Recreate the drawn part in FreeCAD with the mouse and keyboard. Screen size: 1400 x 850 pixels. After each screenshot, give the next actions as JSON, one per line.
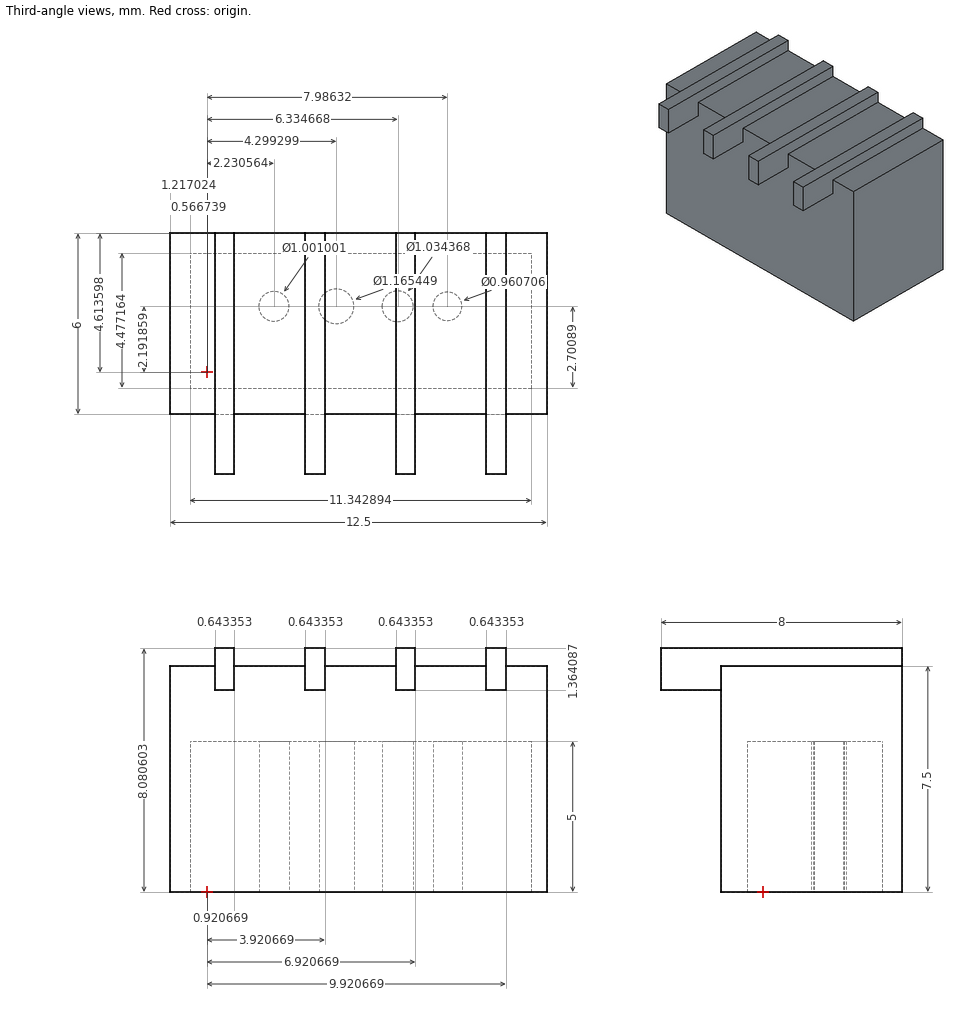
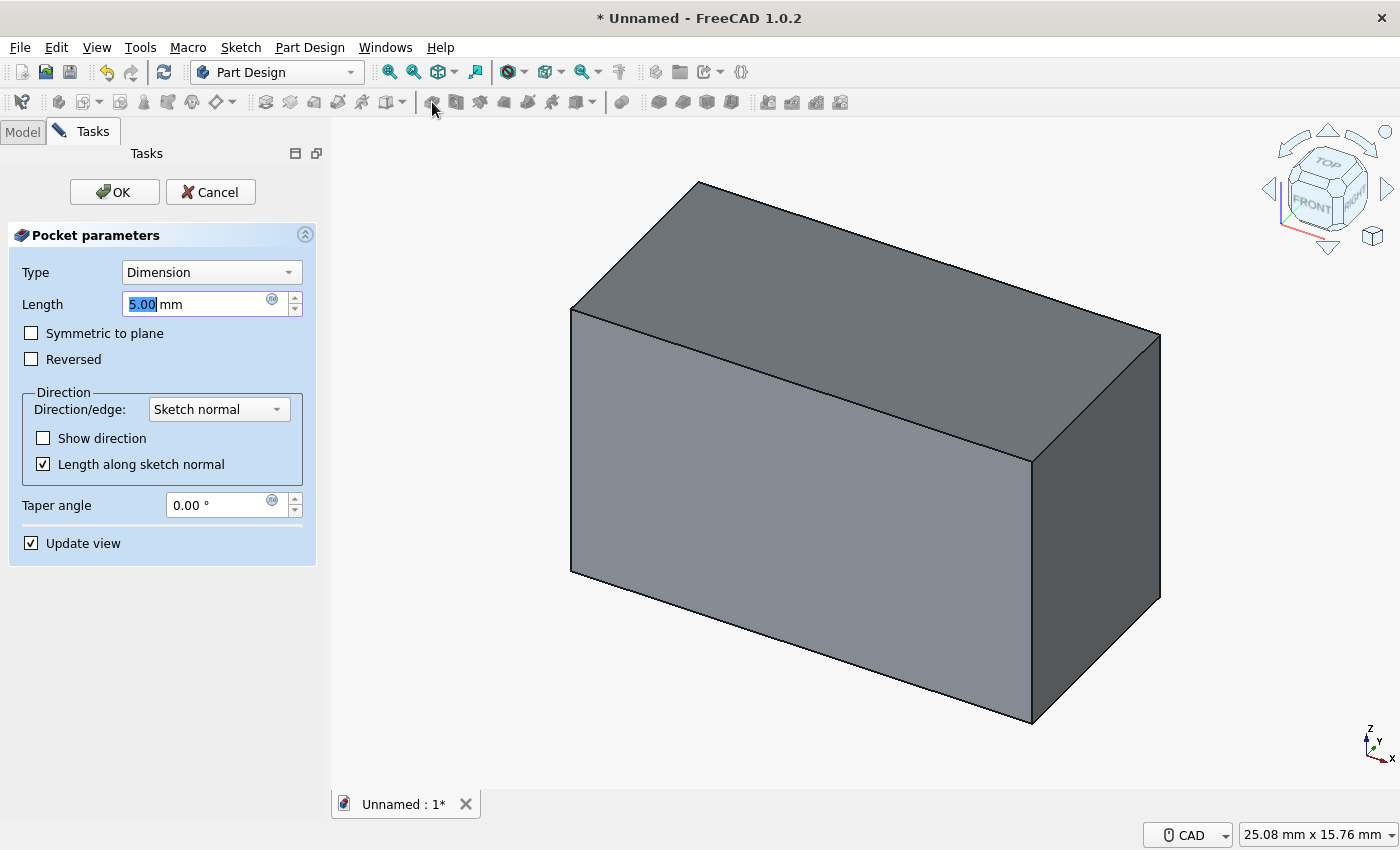
{"action": "type", "text": "5"}
{"action": "key", "text": "Tab"}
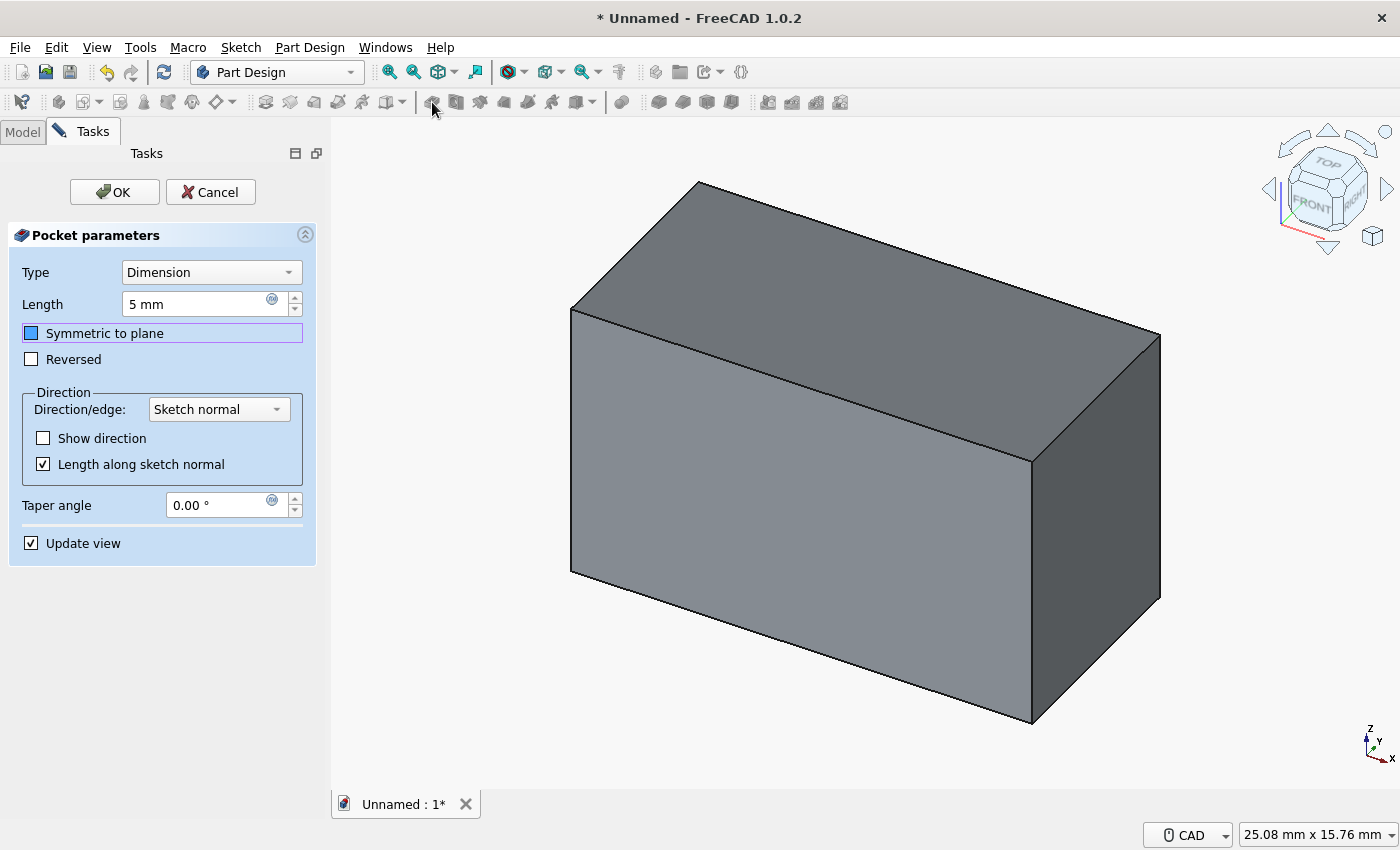
{"action": "left_click", "coordinate": [30, 359]}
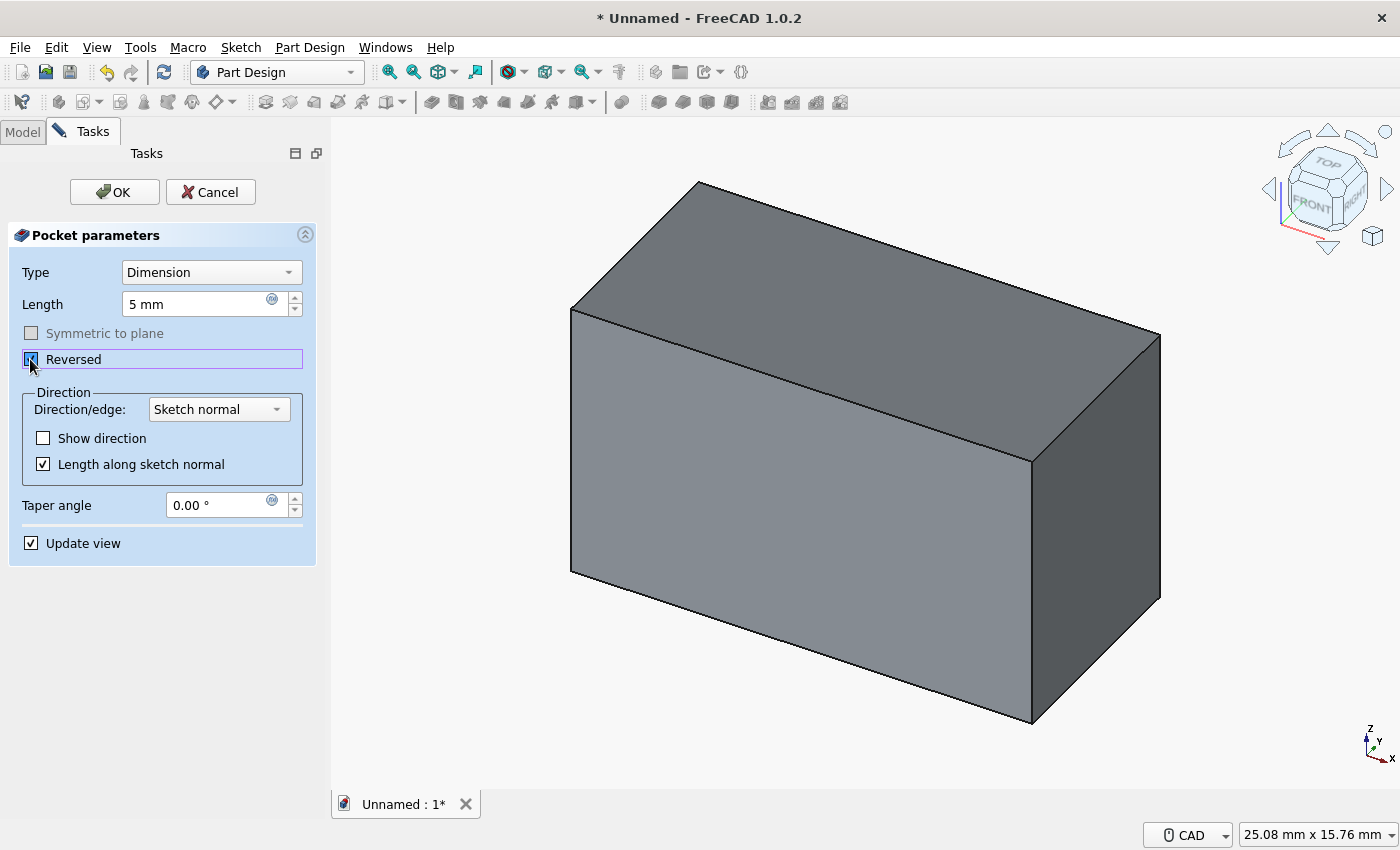
{"action": "left_click", "coordinate": [115, 192]}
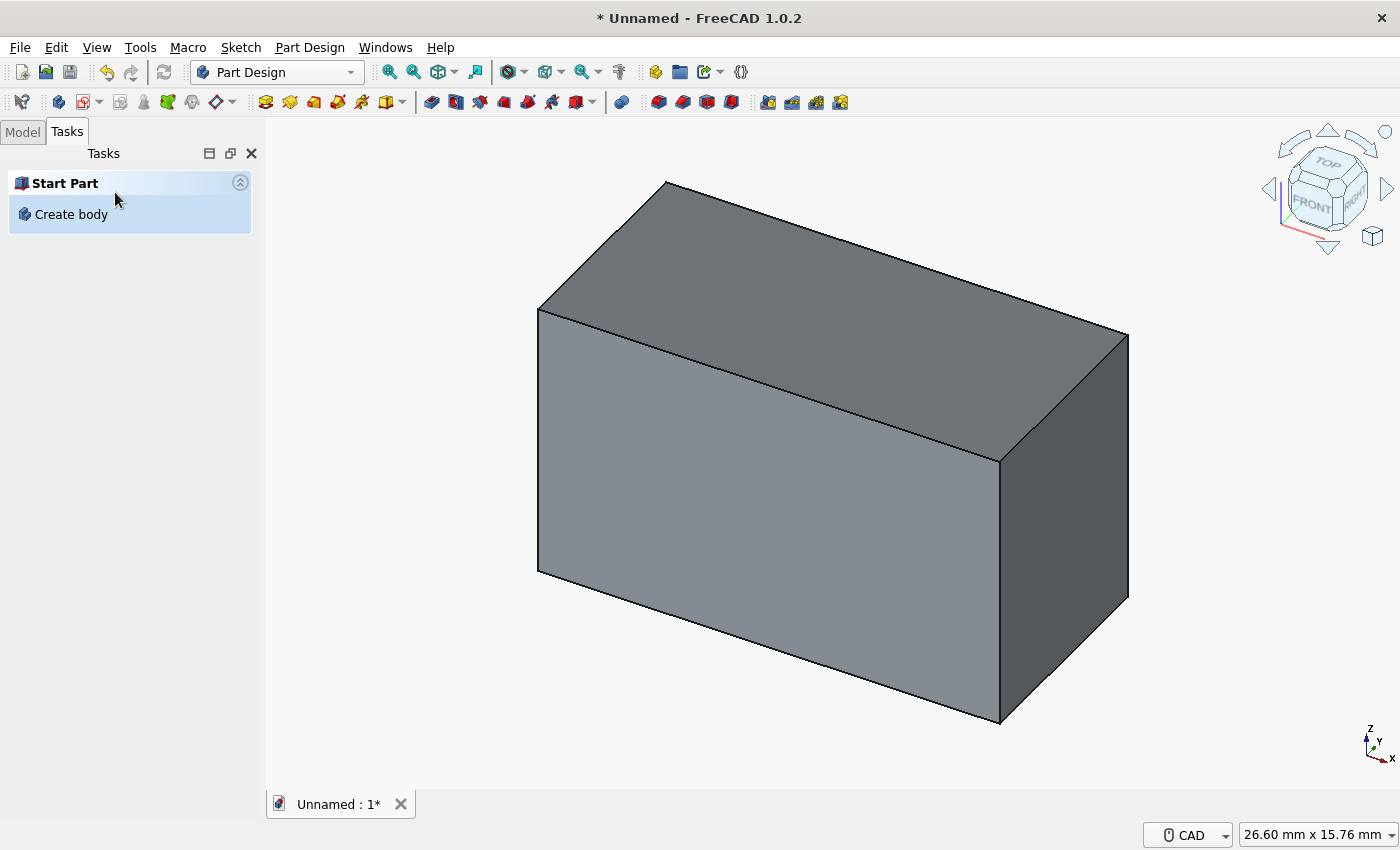
{"action": "key", "text": "4"}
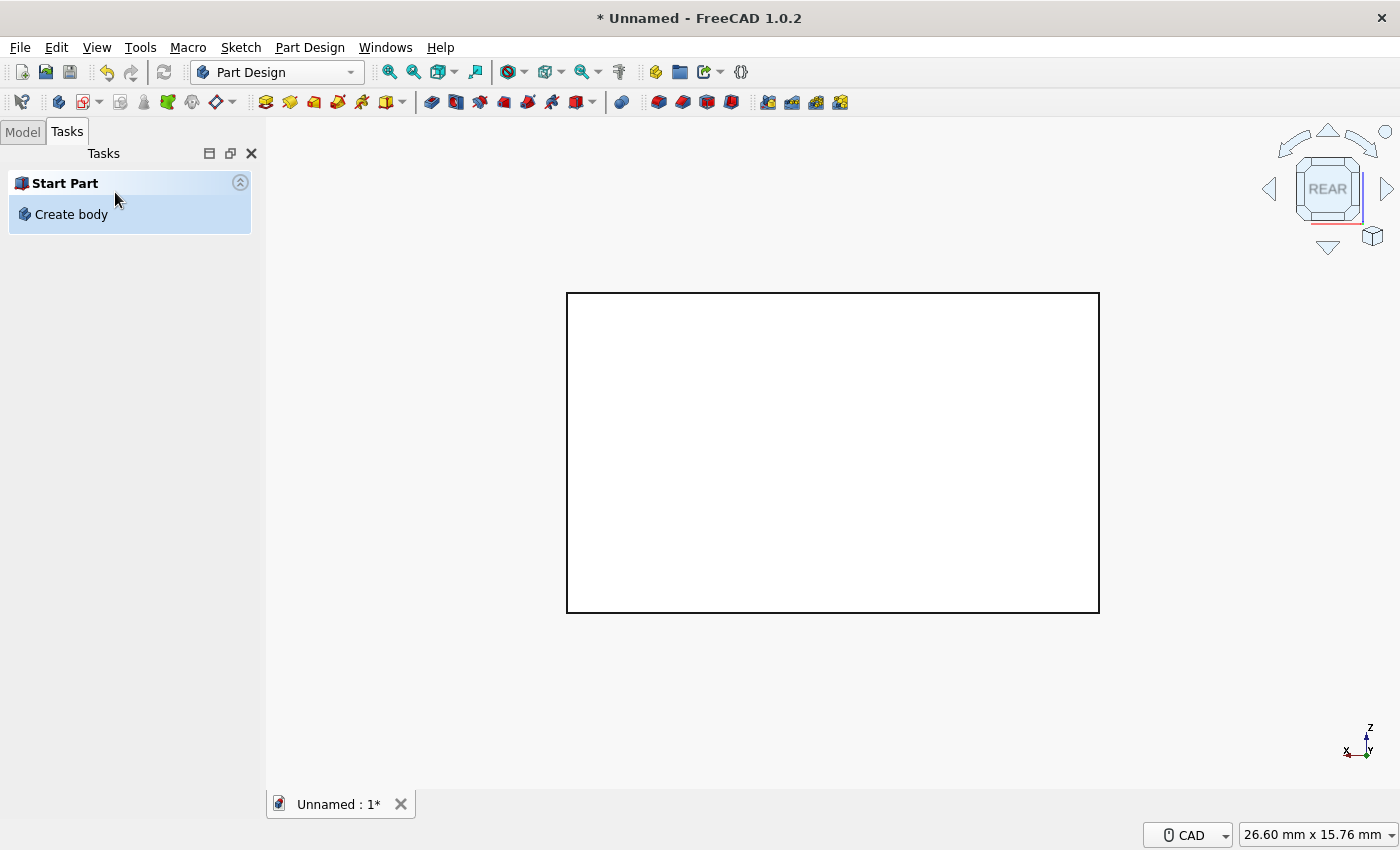
{"action": "left_click", "coordinate": [757, 452]}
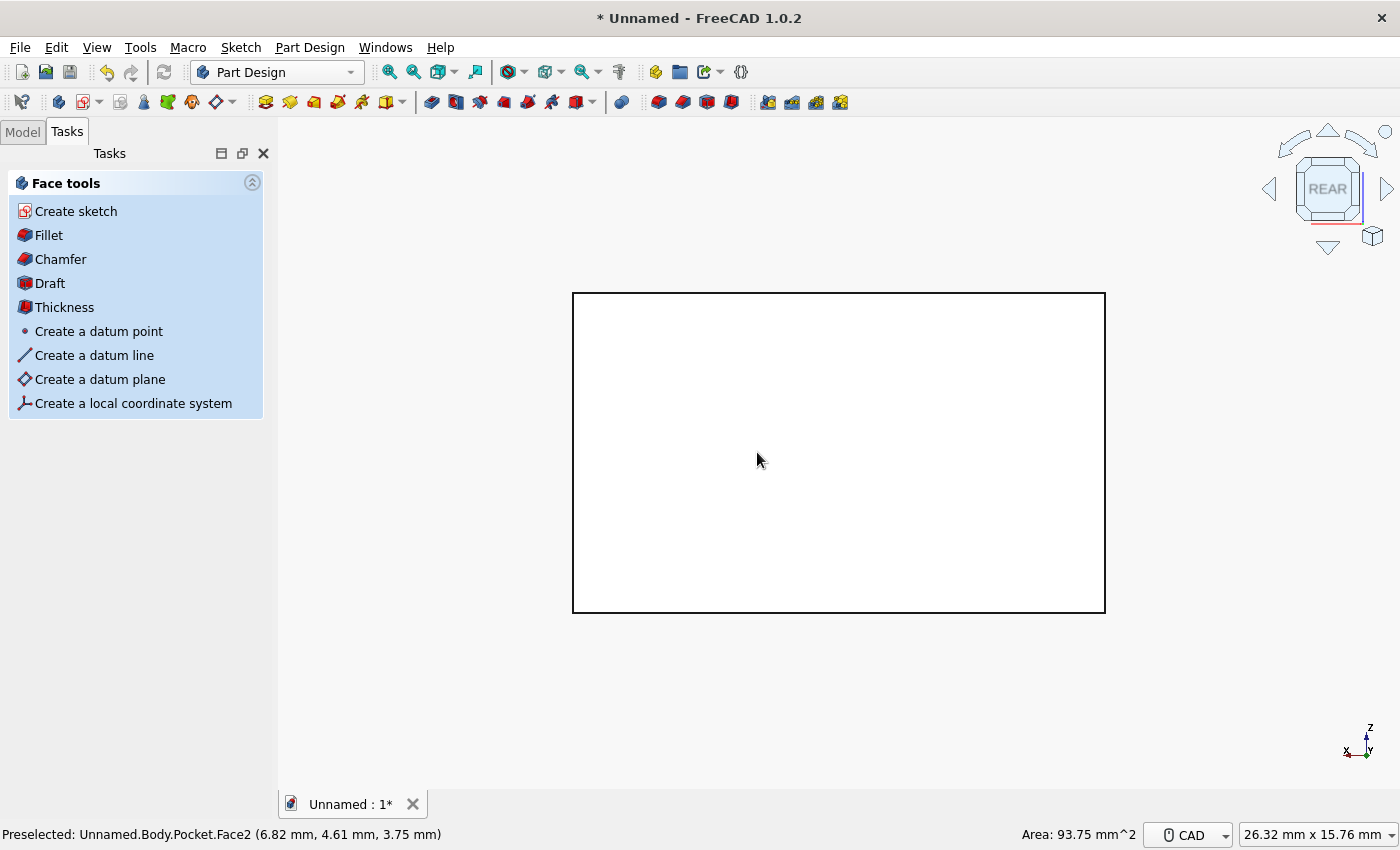
{"action": "left_click", "coordinate": [84, 102]}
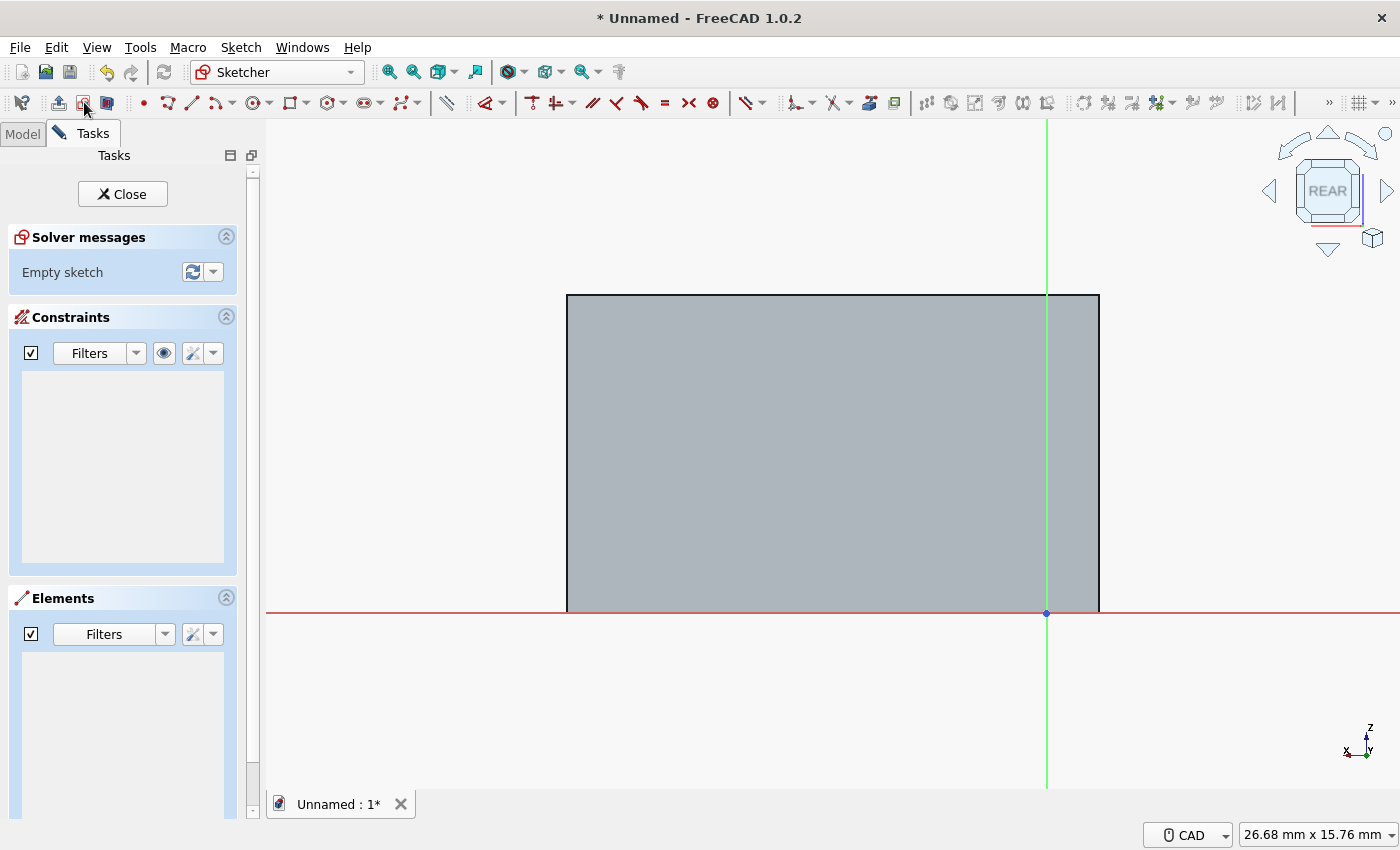
{"action": "key", "text": "g r"}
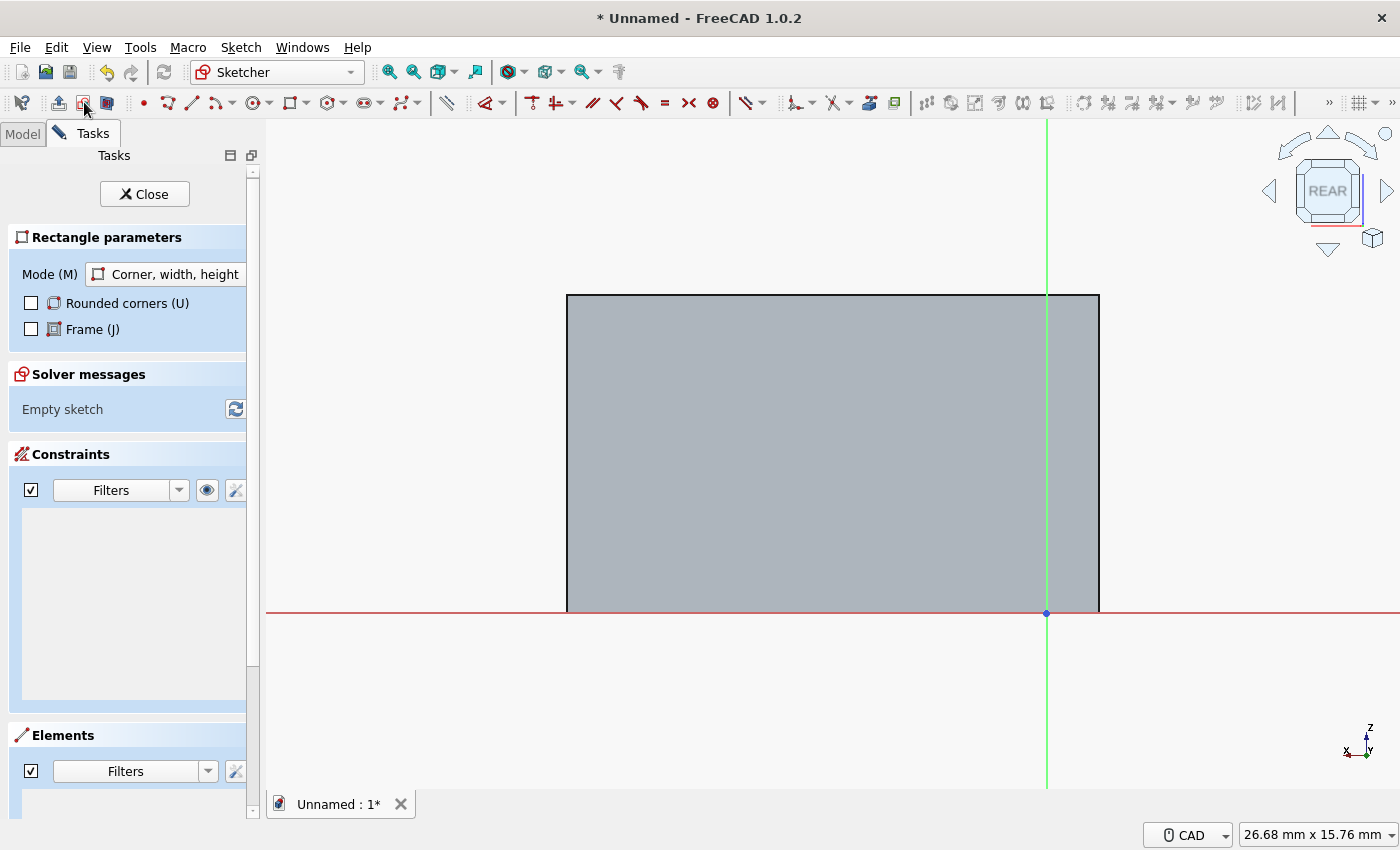
{"action": "left_click", "coordinate": [753, 270]}
{"action": "left_click", "coordinate": [780, 328]}